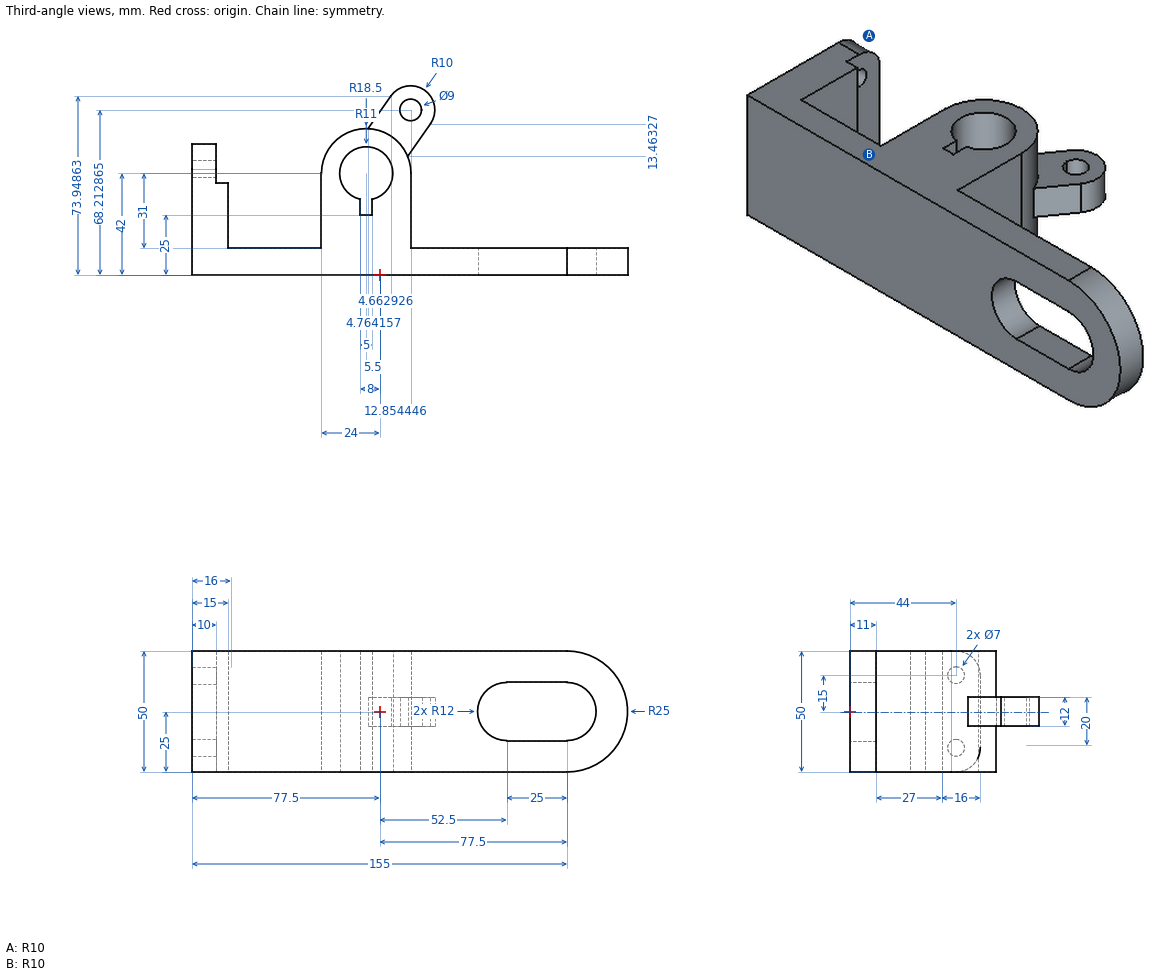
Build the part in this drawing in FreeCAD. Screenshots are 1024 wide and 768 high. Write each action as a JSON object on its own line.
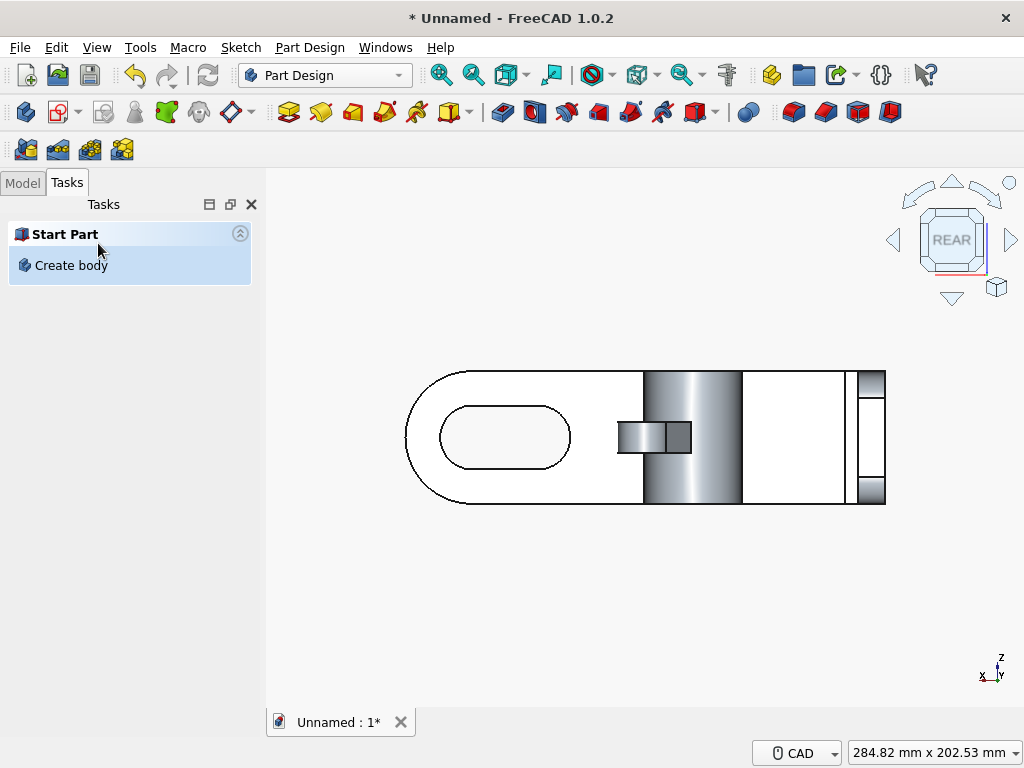
{"action": "key", "text": "6"}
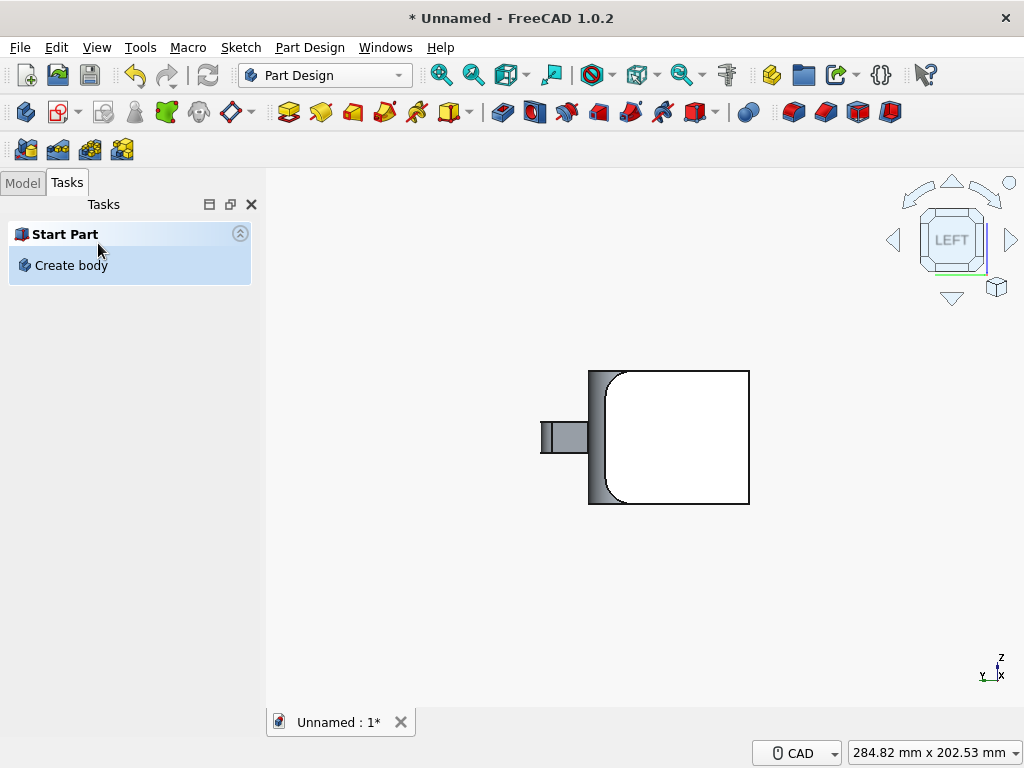
{"action": "key", "text": "v f"}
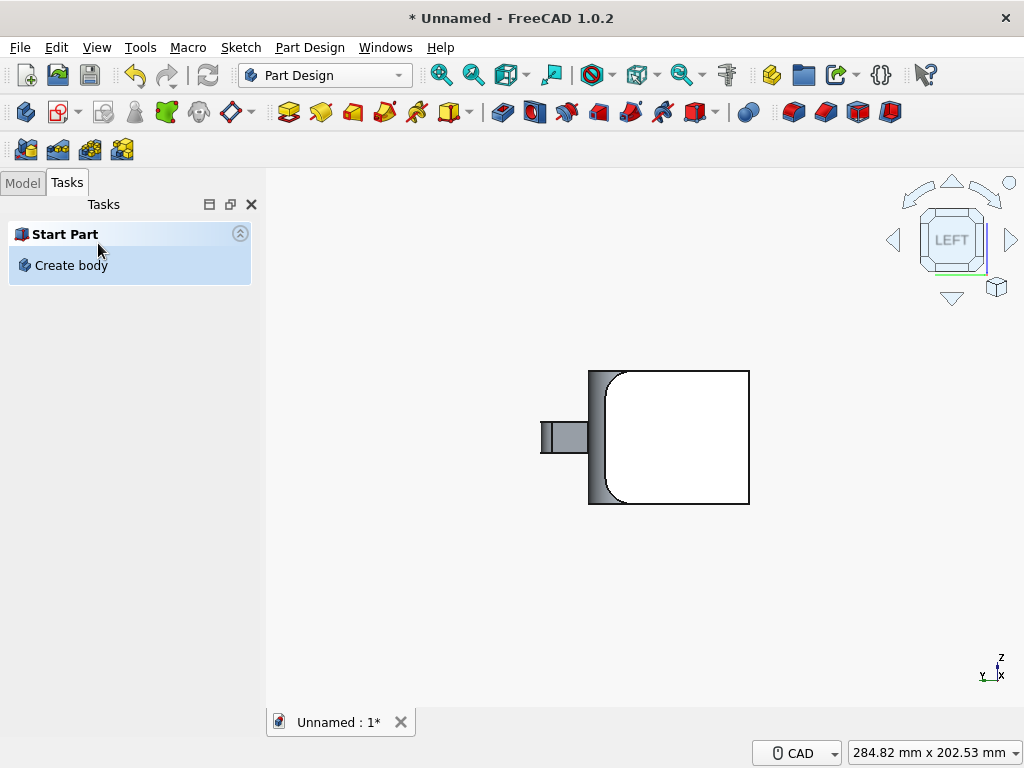
{"action": "left_click", "coordinate": [677, 437]}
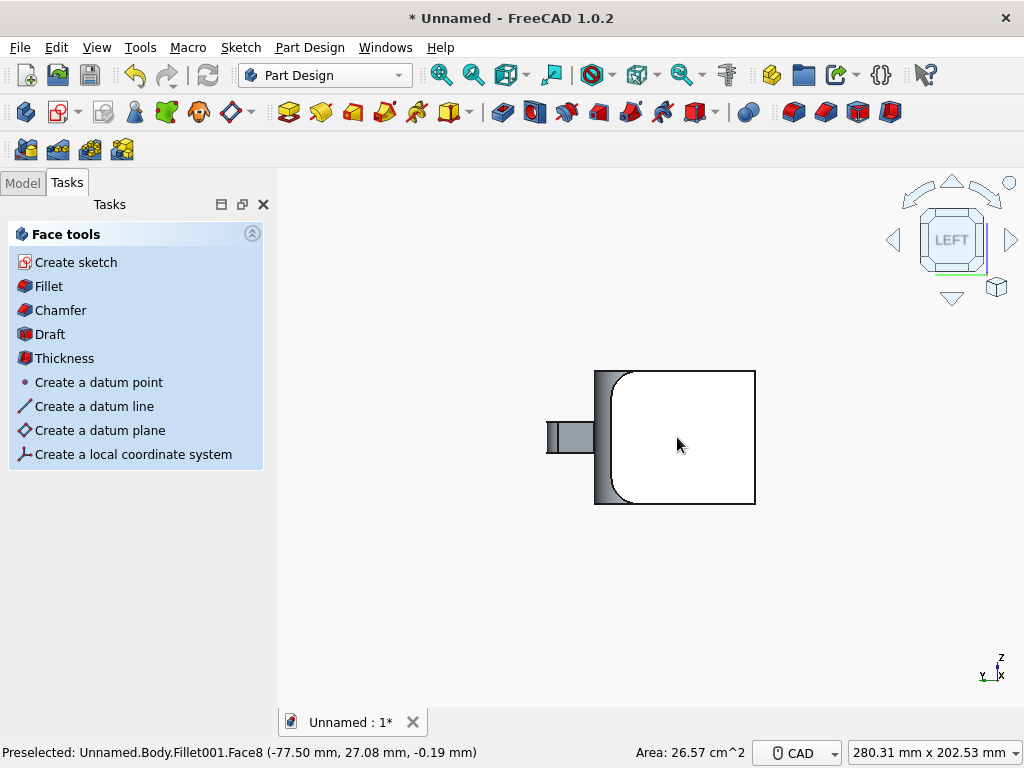
{"action": "left_click", "coordinate": [58, 112]}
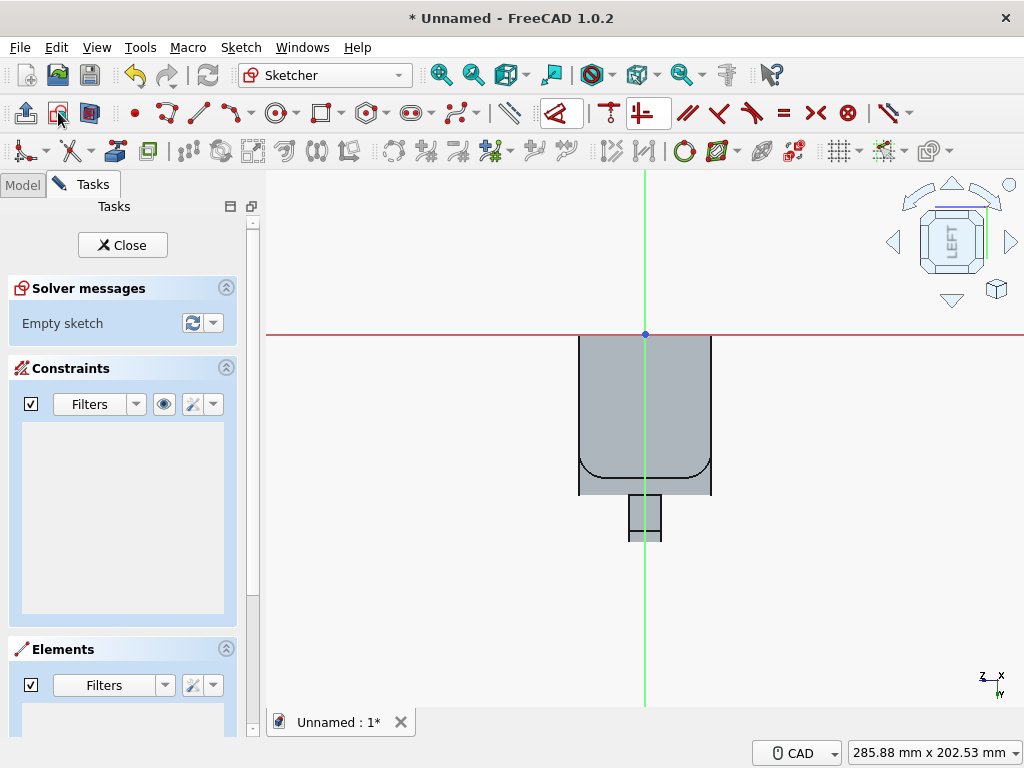
{"action": "scroll", "coordinate": [685, 374], "scroll_direction": "up", "scroll_amount": 5}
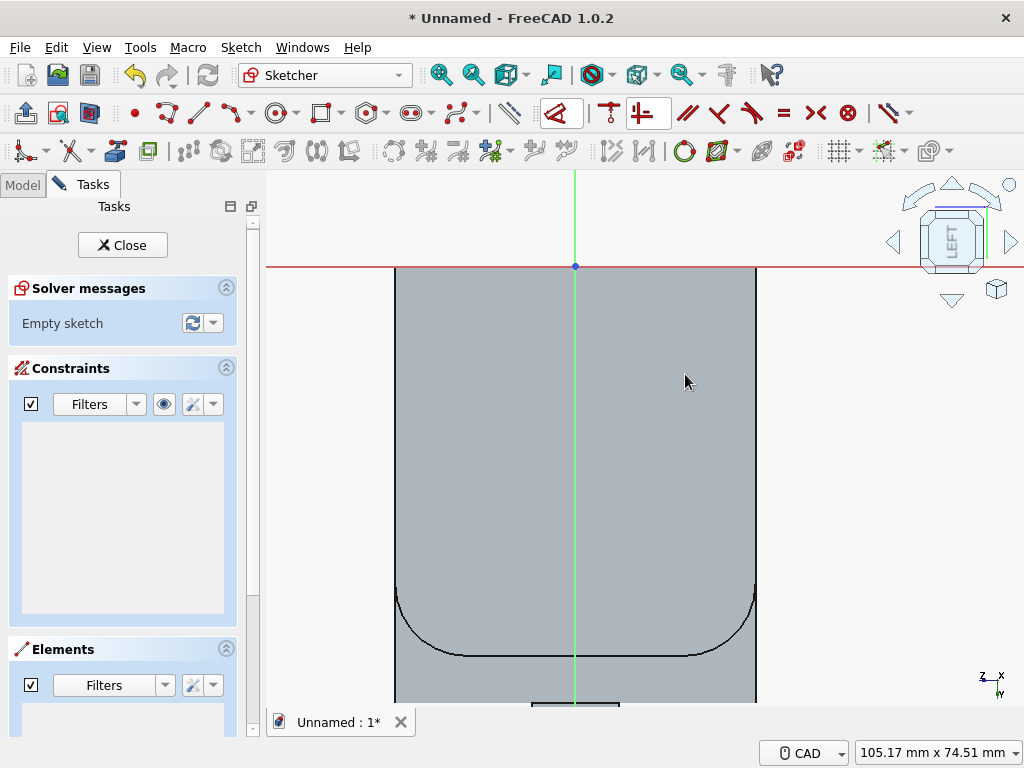
{"action": "left_click", "coordinate": [276, 114]}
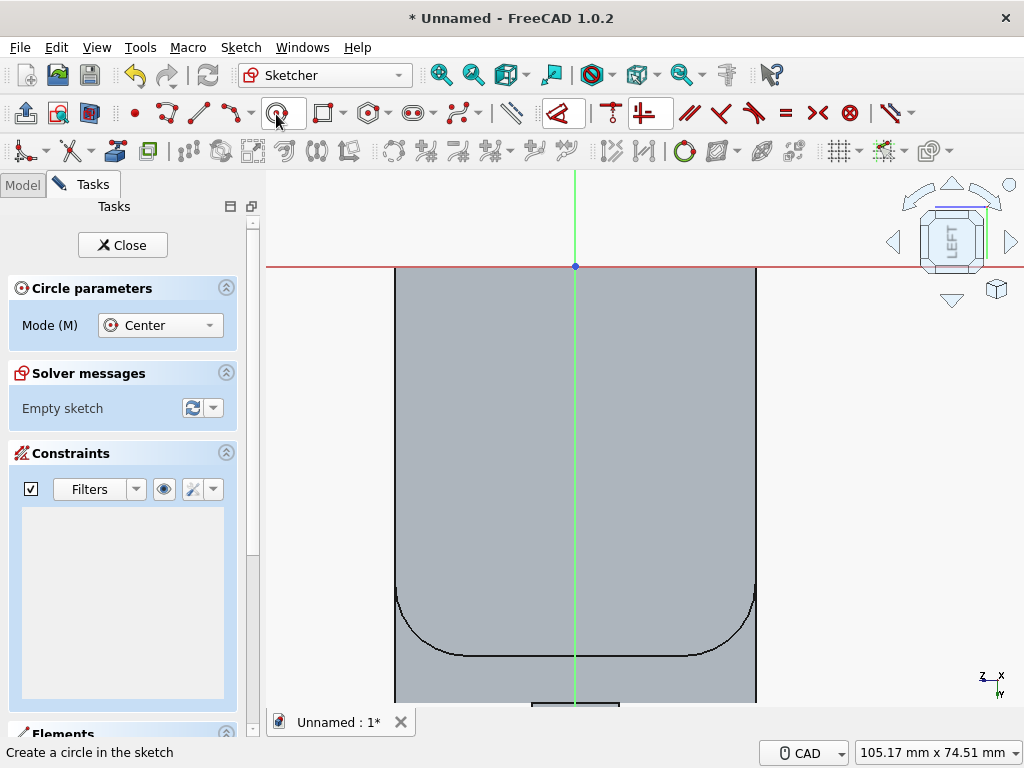
{"action": "left_click", "coordinate": [467, 584]}
{"action": "left_click", "coordinate": [485, 566]}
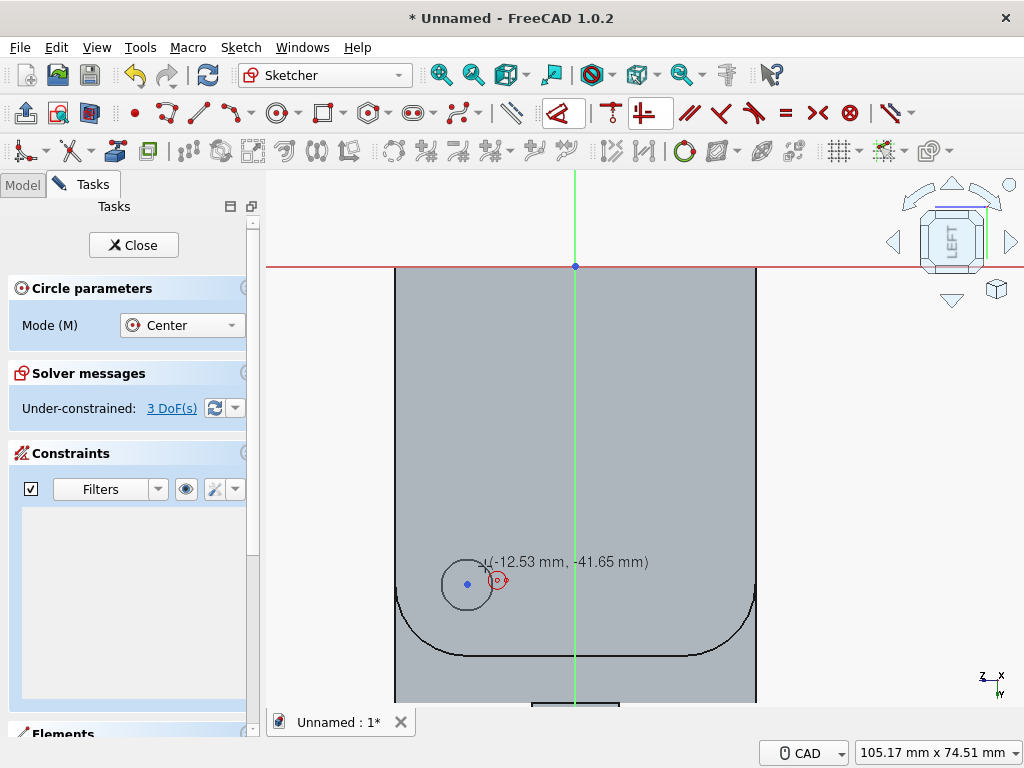
{"action": "left_click", "coordinate": [683, 584]}
{"action": "left_click", "coordinate": [701, 566]}
{"action": "key", "text": "Escape"}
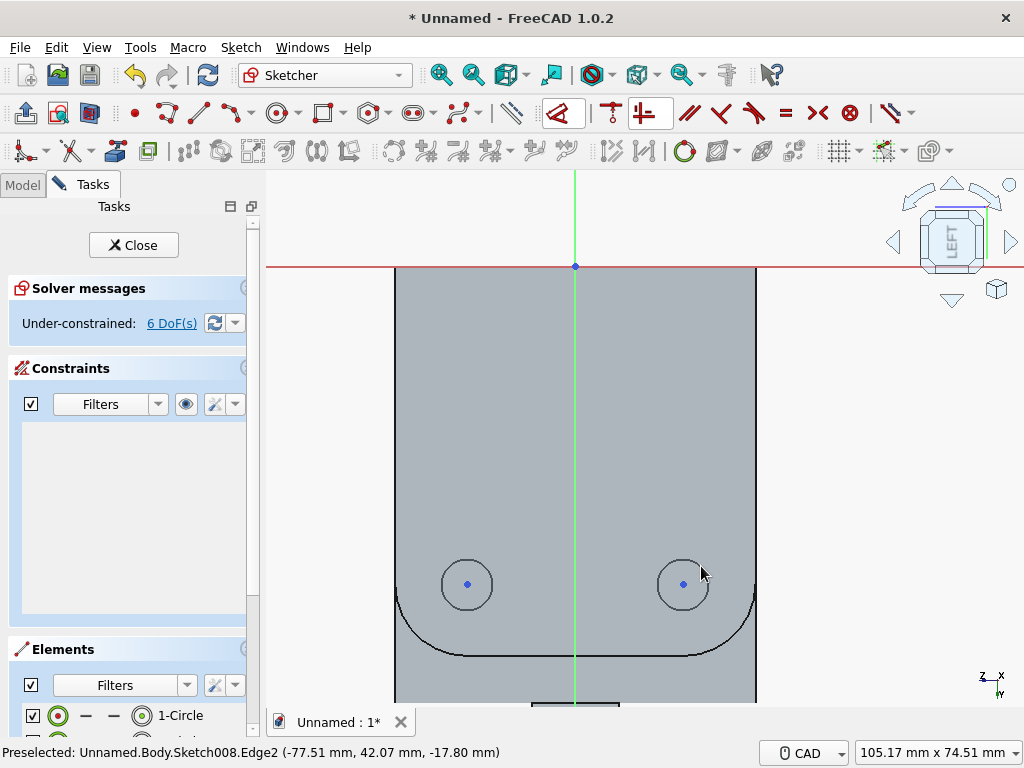
{"action": "left_click", "coordinate": [485, 567]}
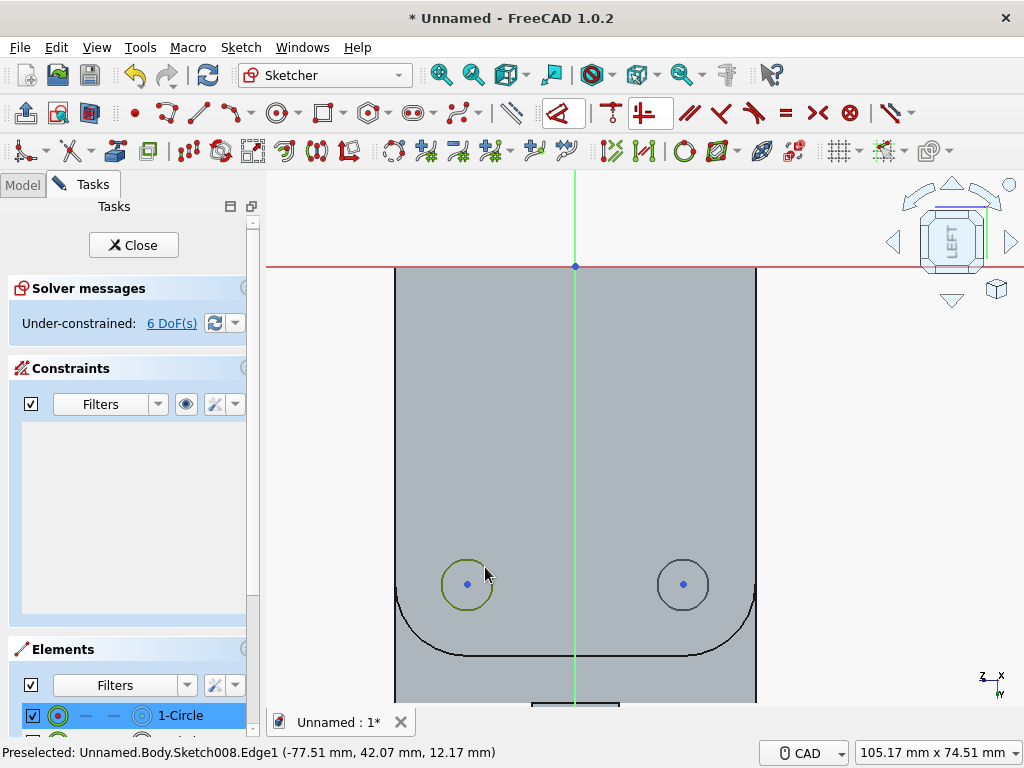
{"action": "left_click", "coordinate": [701, 567]}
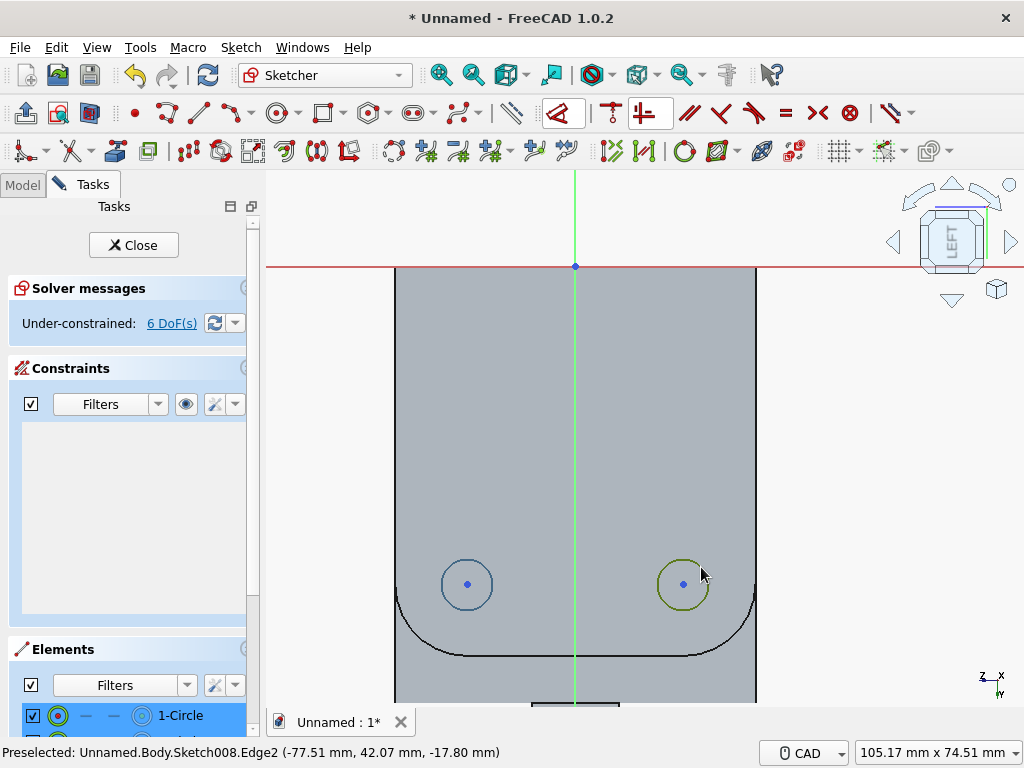
{"action": "left_click", "coordinate": [786, 114]}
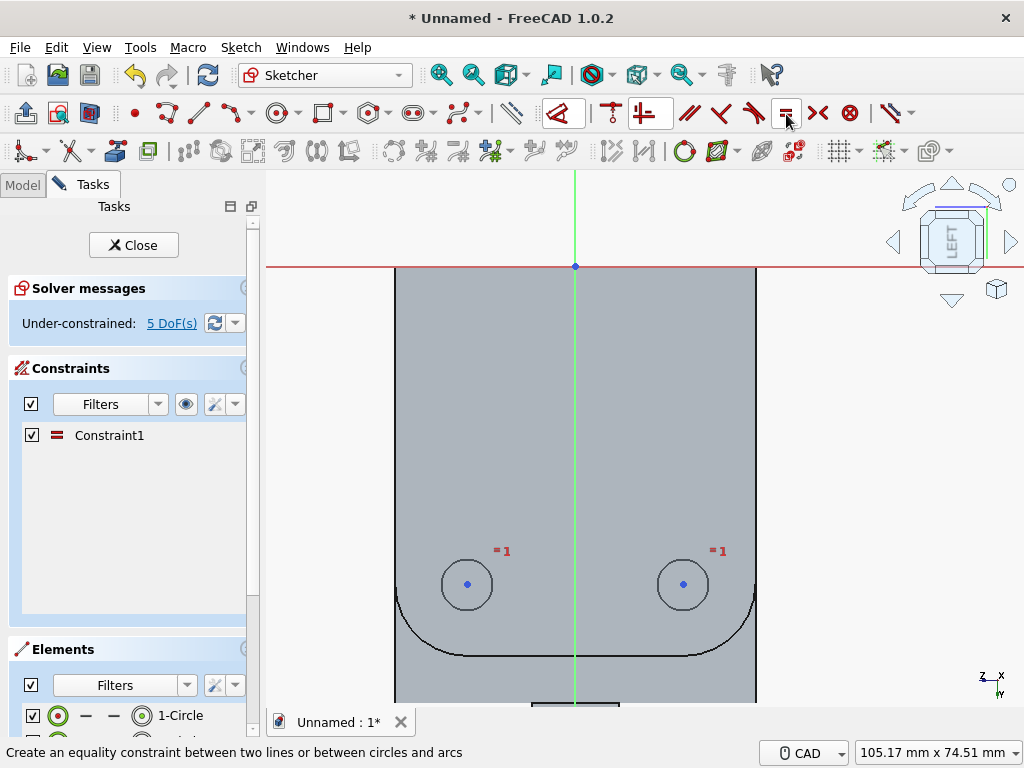
{"action": "left_click", "coordinate": [467, 585]}